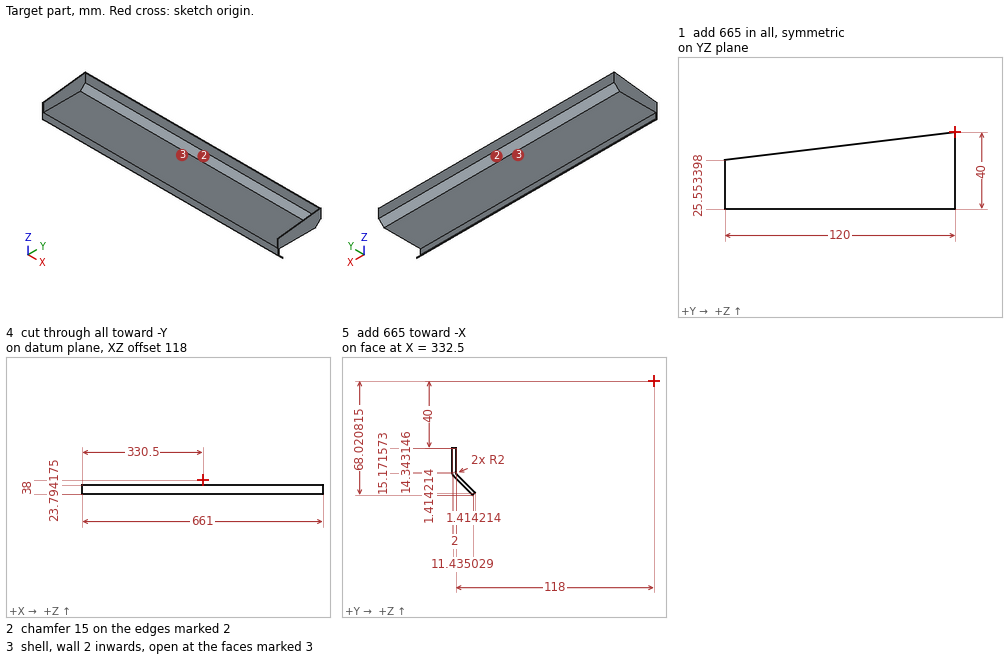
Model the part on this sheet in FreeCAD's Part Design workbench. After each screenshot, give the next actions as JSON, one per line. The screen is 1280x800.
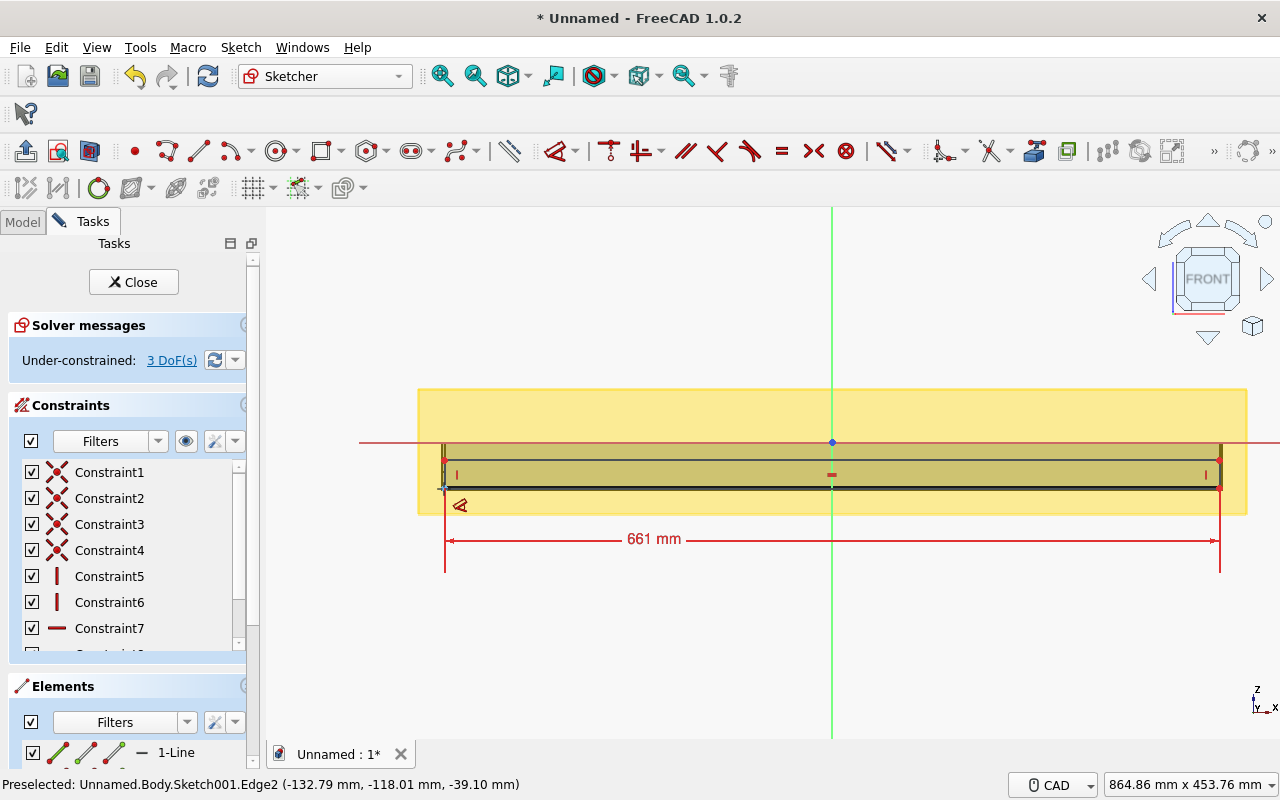
{"action": "left_click", "coordinate": [445, 489]}
{"action": "left_click", "coordinate": [411, 466]}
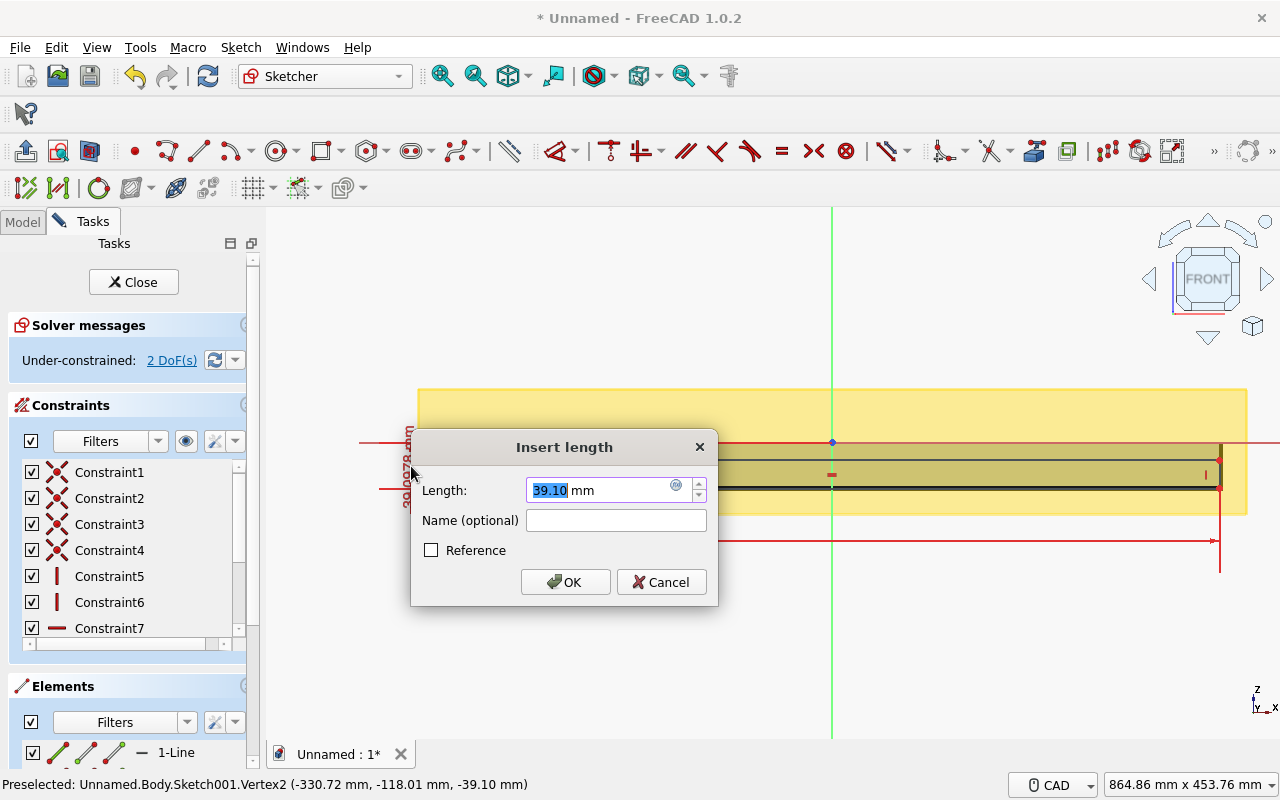
{"action": "type", "text": "38"}
{"action": "key", "text": "Return"}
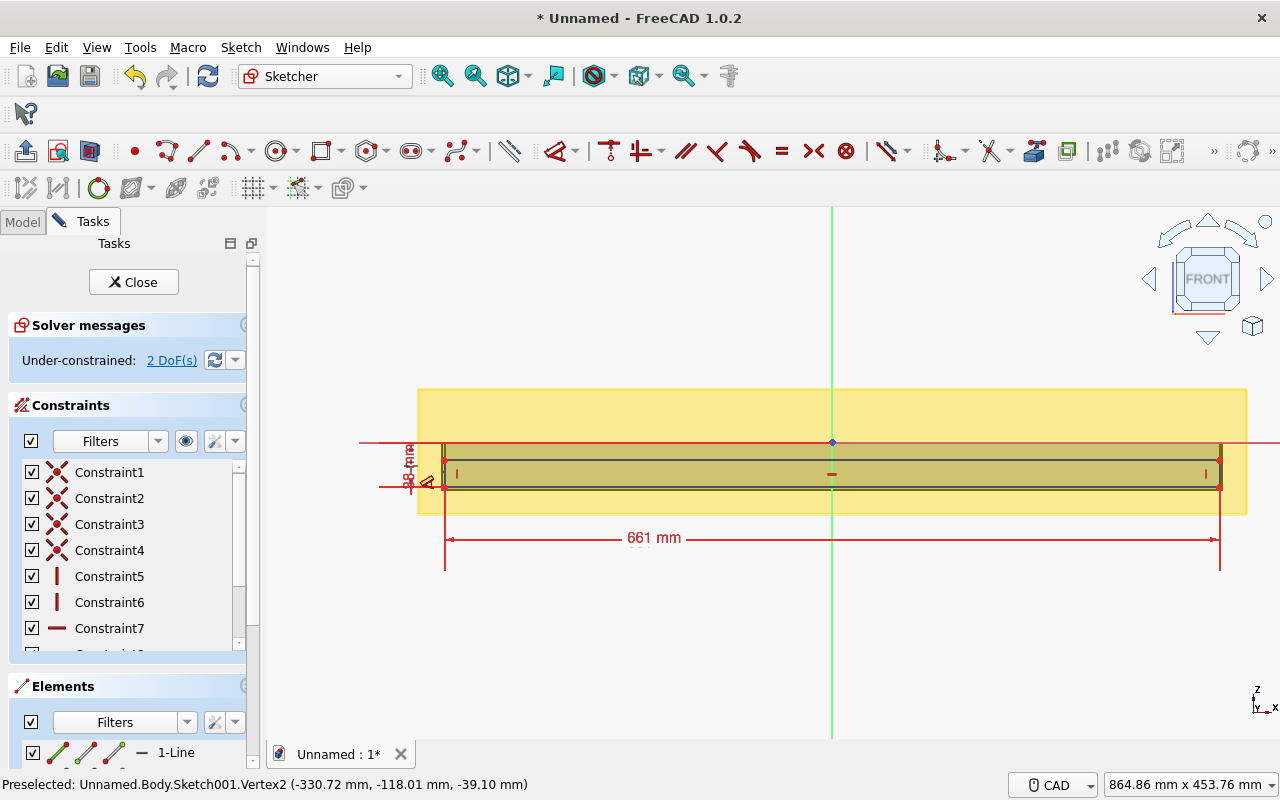
{"action": "left_click", "coordinate": [445, 460]}
{"action": "left_click", "coordinate": [638, 409]}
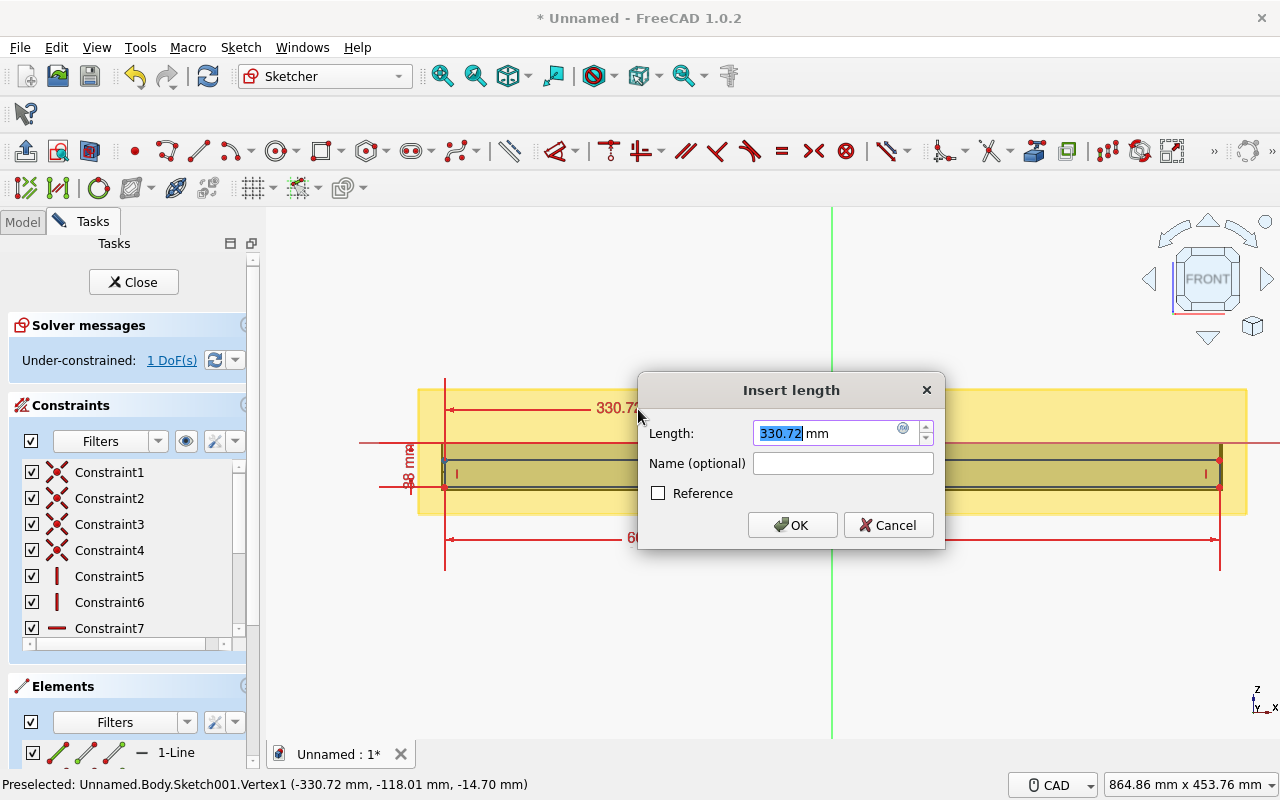
{"action": "type", "text": "330.5"}
{"action": "key", "text": "Return"}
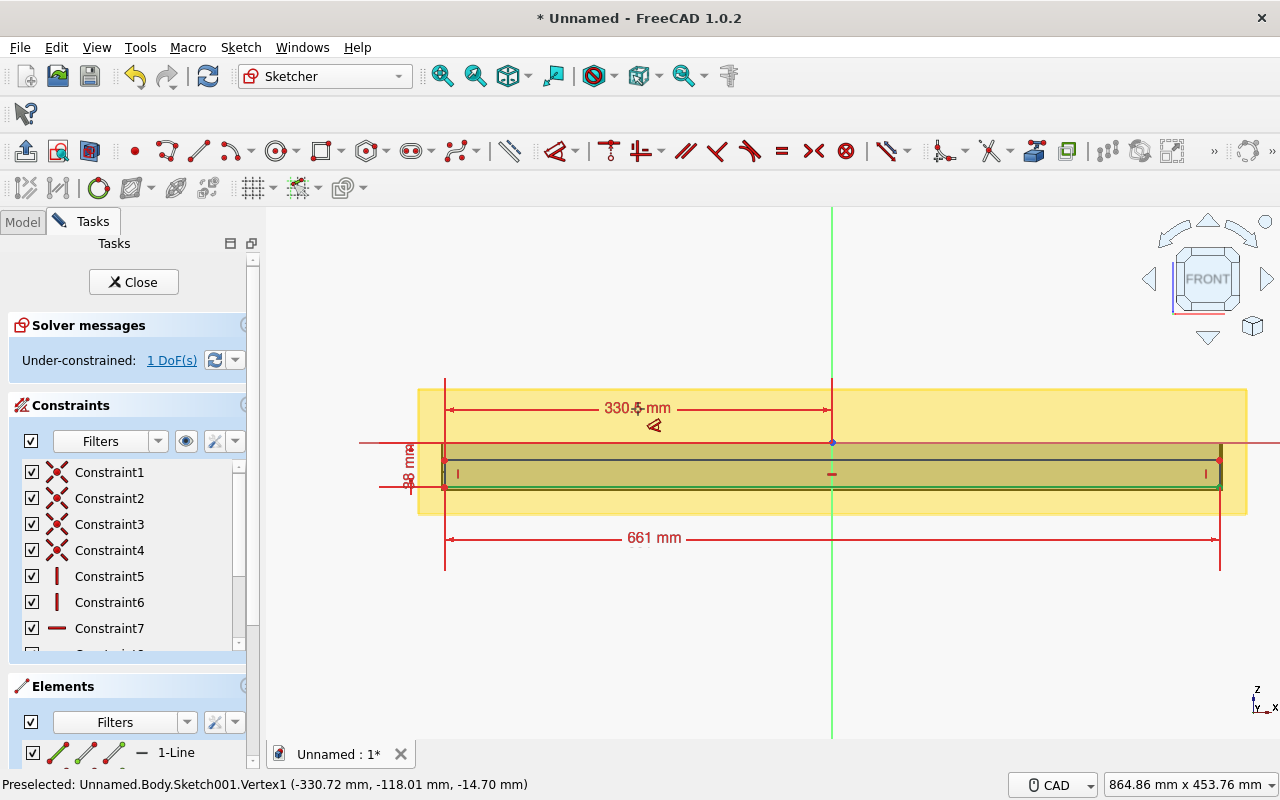
{"action": "scroll", "coordinate": [445, 471], "scroll_direction": "up", "scroll_amount": 2}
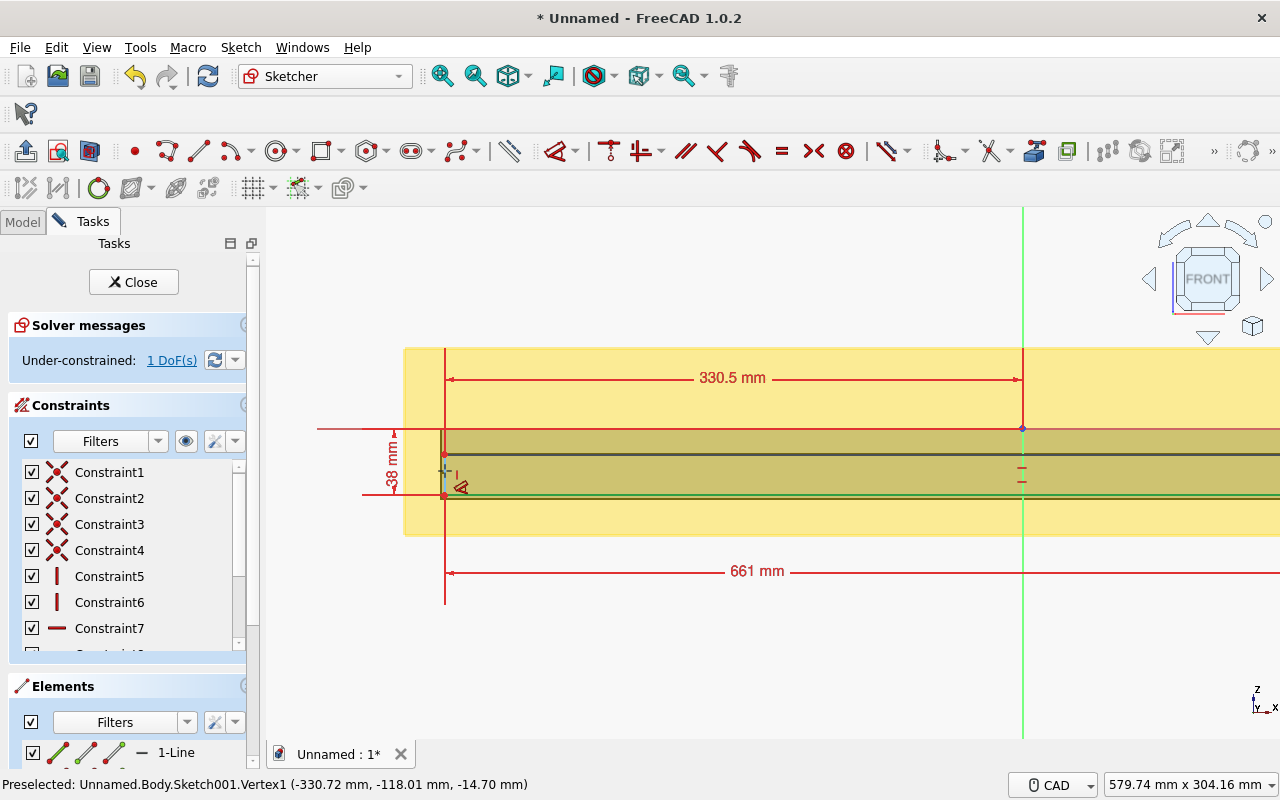
{"action": "left_click", "coordinate": [445, 471]}
{"action": "left_click", "coordinate": [411, 484]}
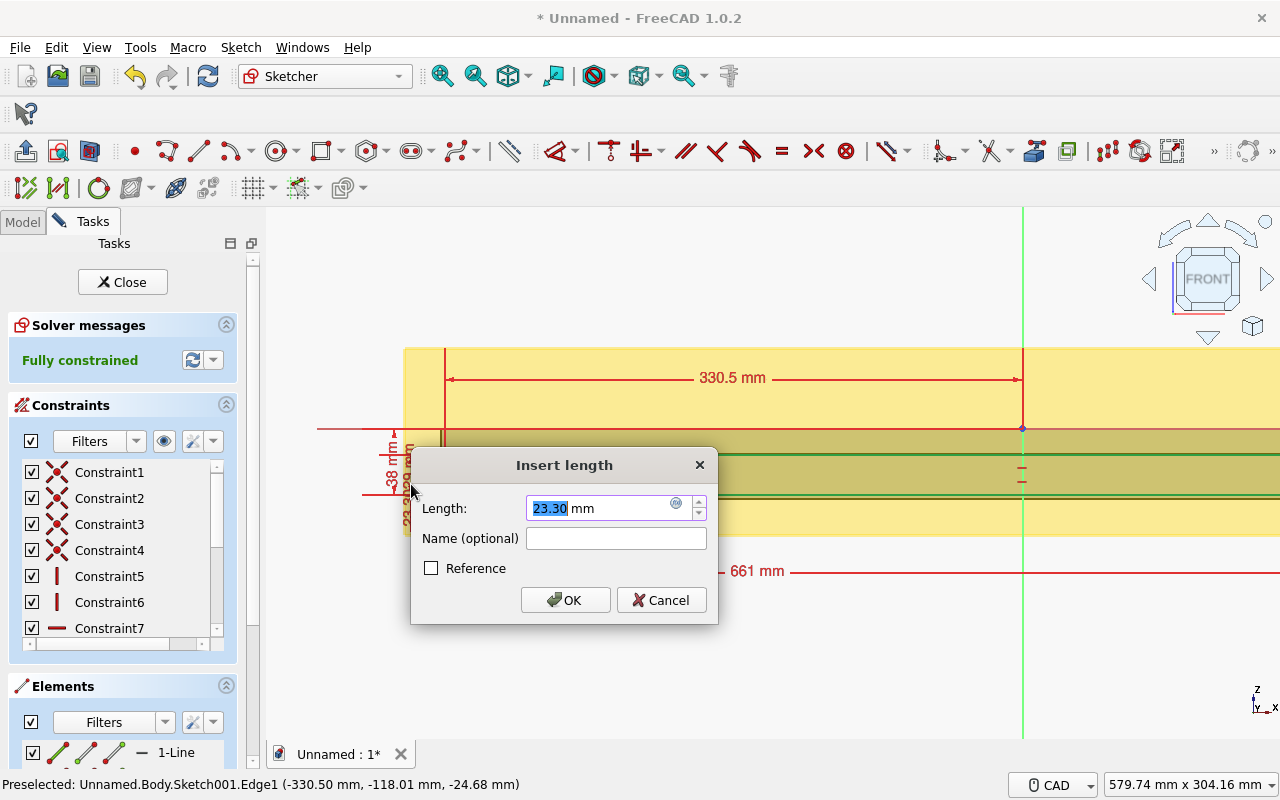
{"action": "type", "text": "23.794175"}
{"action": "key", "text": "Return"}
{"action": "key", "text": "Escape"}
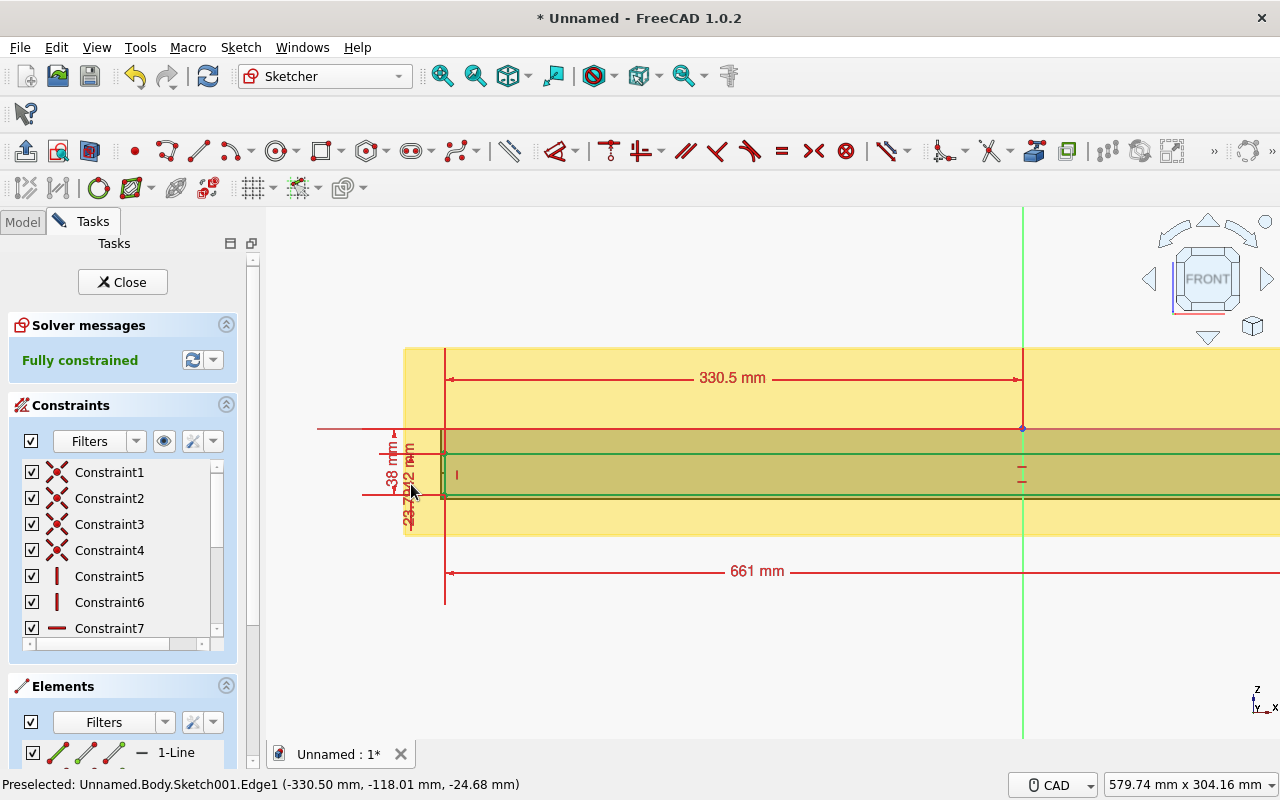
{"action": "left_click", "coordinate": [123, 282]}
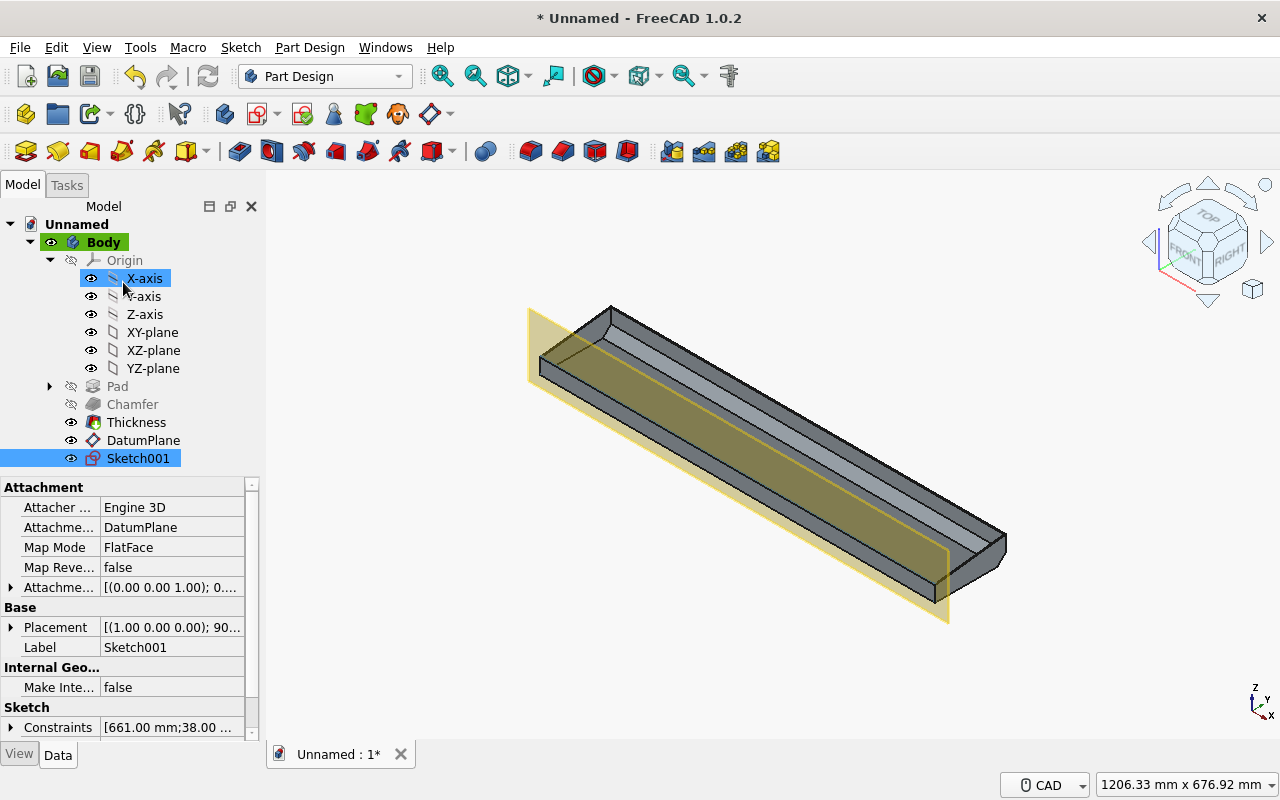
{"action": "left_click", "coordinate": [240, 152]}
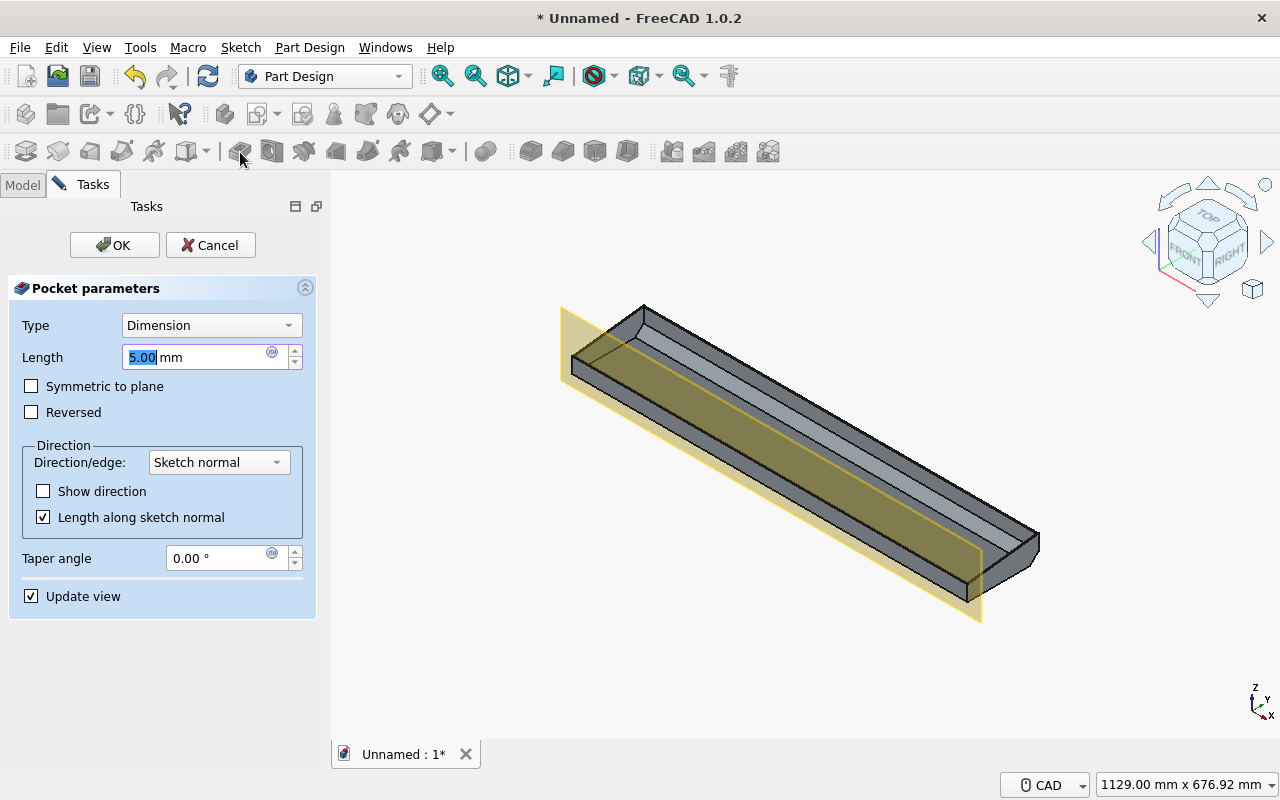
{"action": "left_click", "coordinate": [212, 326]}